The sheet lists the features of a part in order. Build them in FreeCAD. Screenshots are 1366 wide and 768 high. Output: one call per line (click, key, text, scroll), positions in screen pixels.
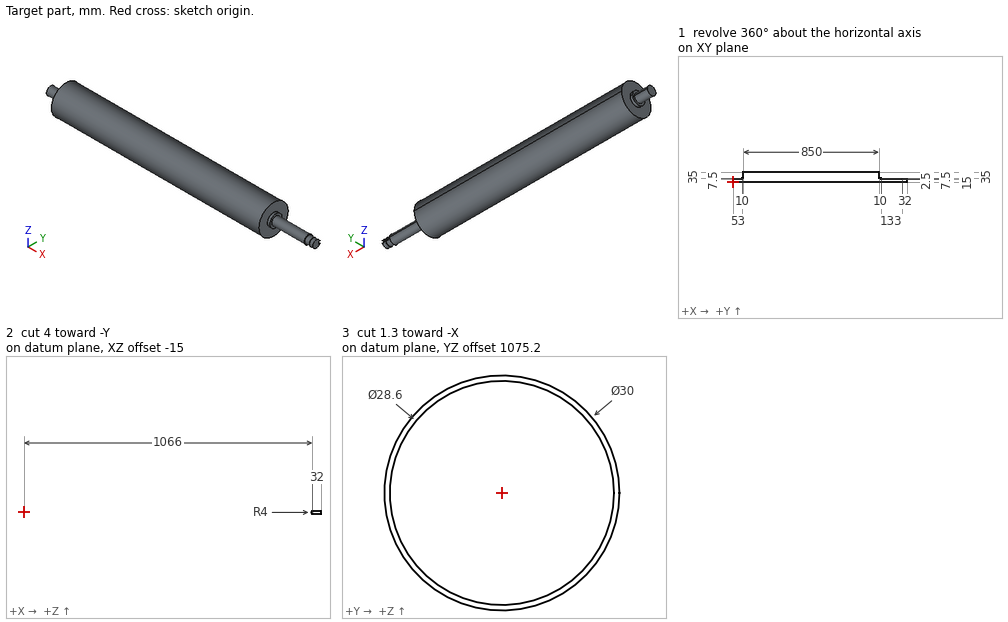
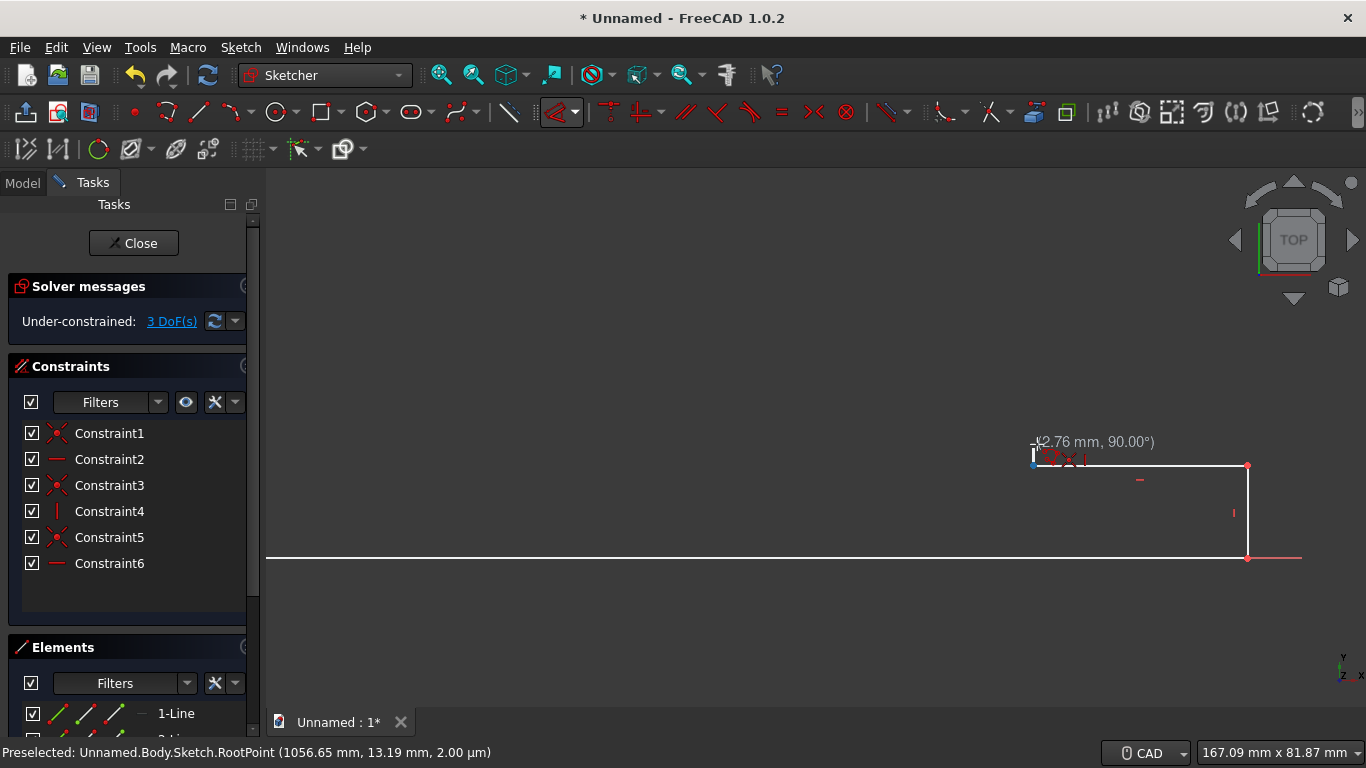
click(1033, 443)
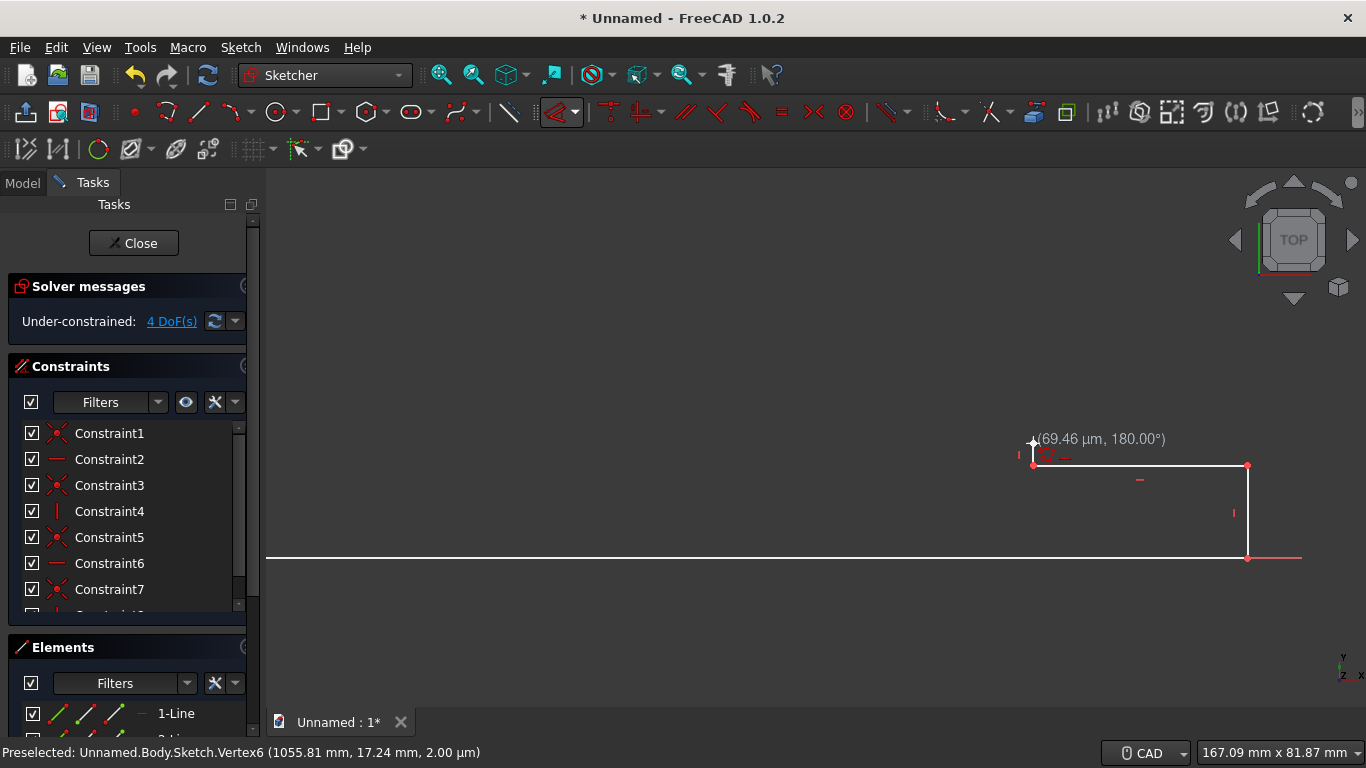
scroll(1055, 445, down, 12)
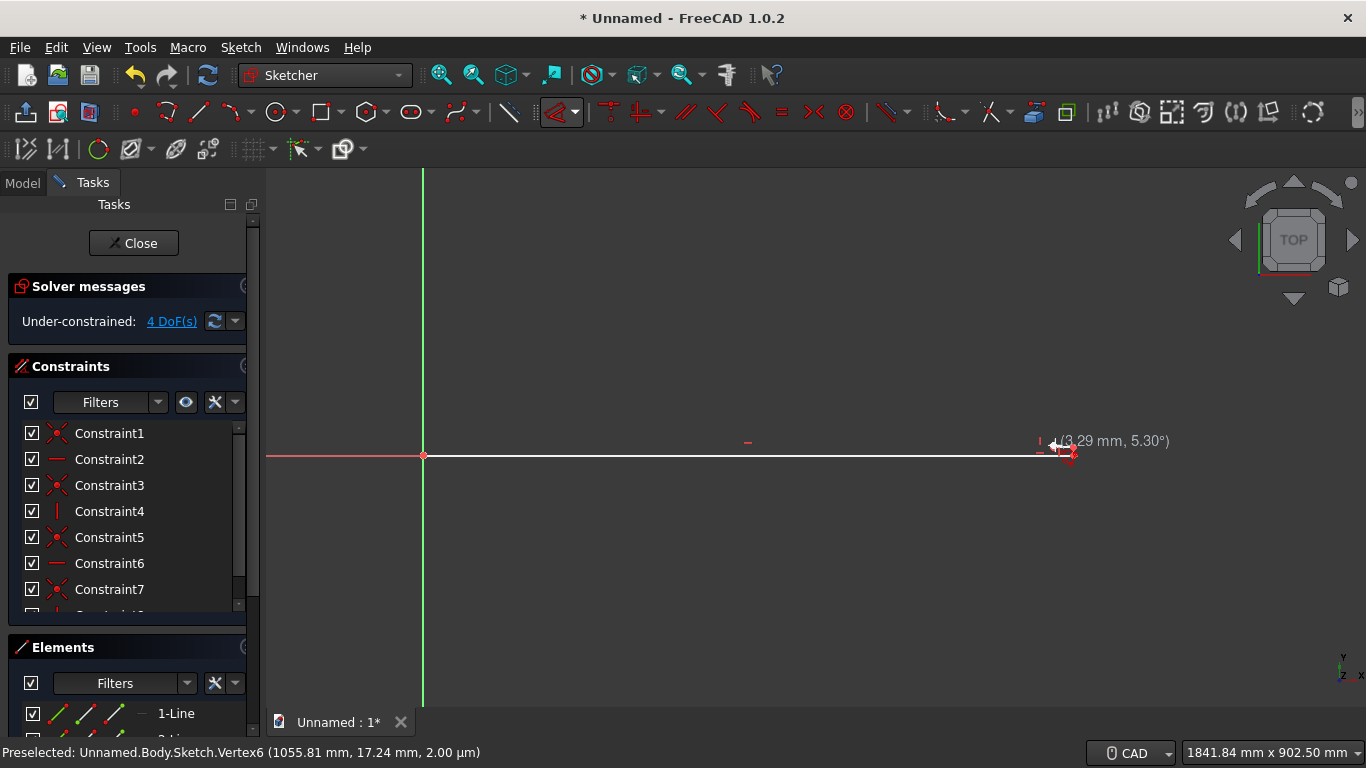
scroll(974, 445, up, 3)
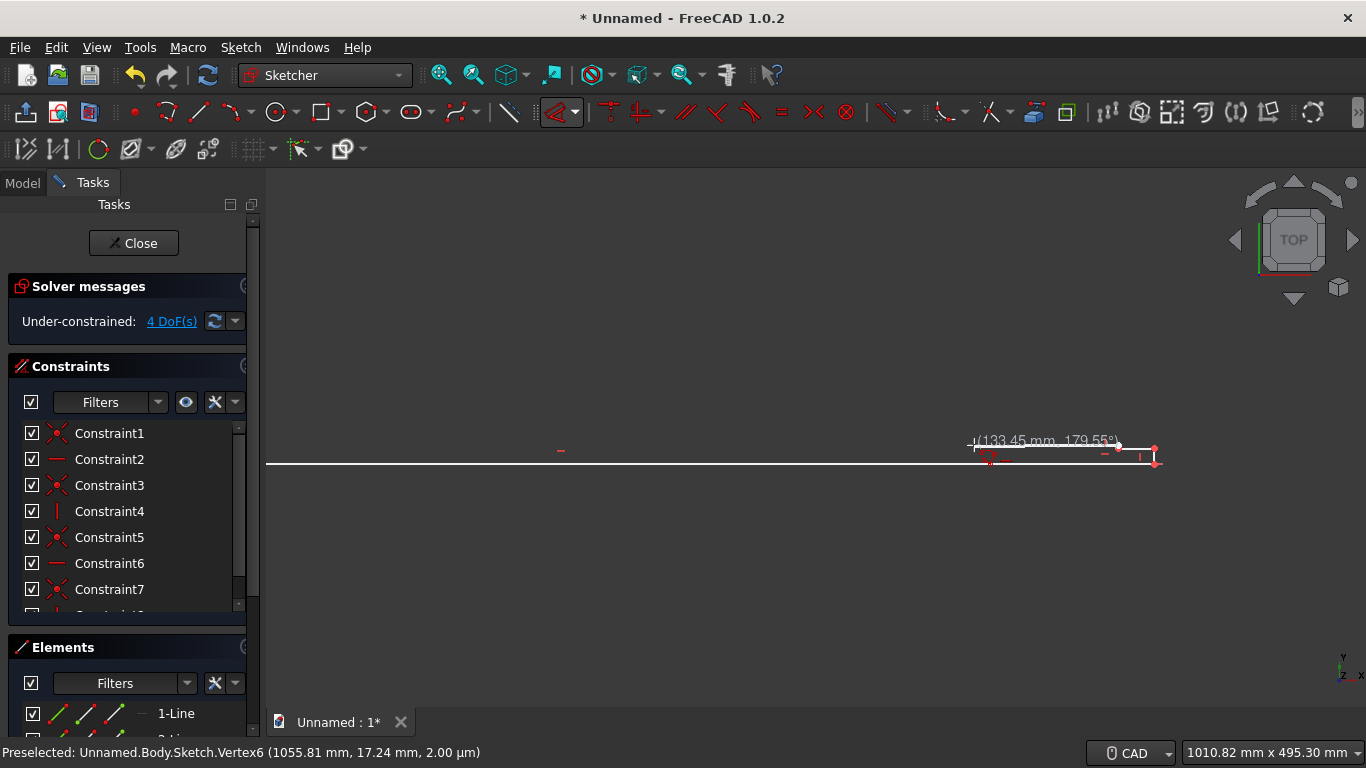
click(974, 445)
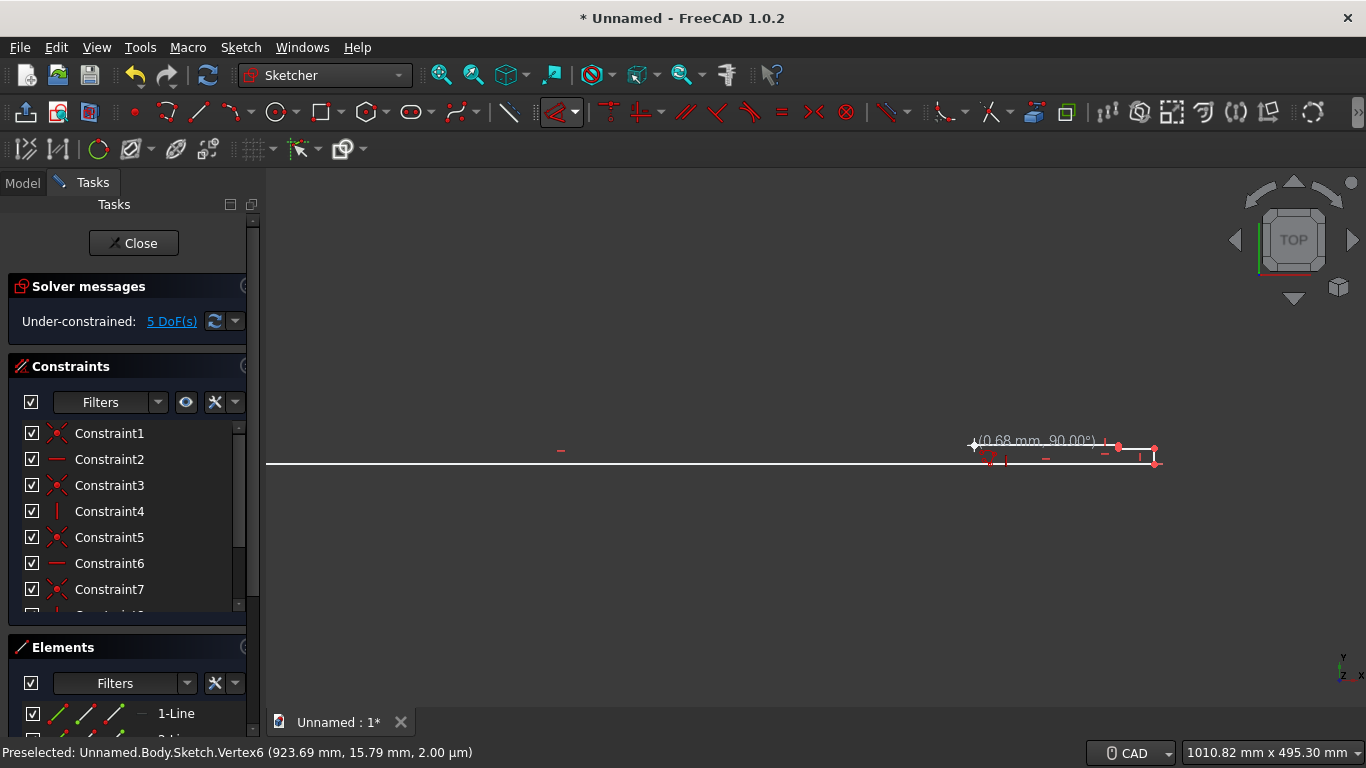
scroll(974, 437, up, 4)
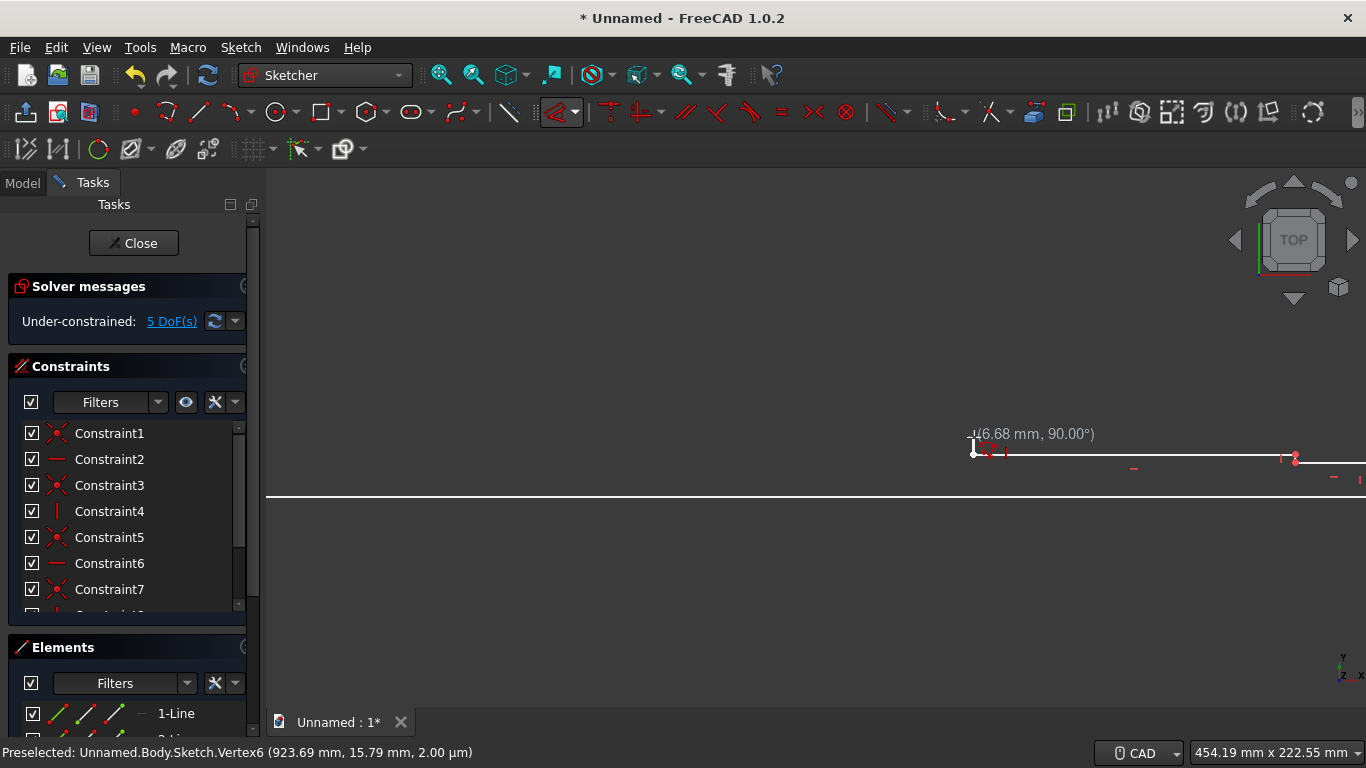
click(973, 436)
click(950, 436)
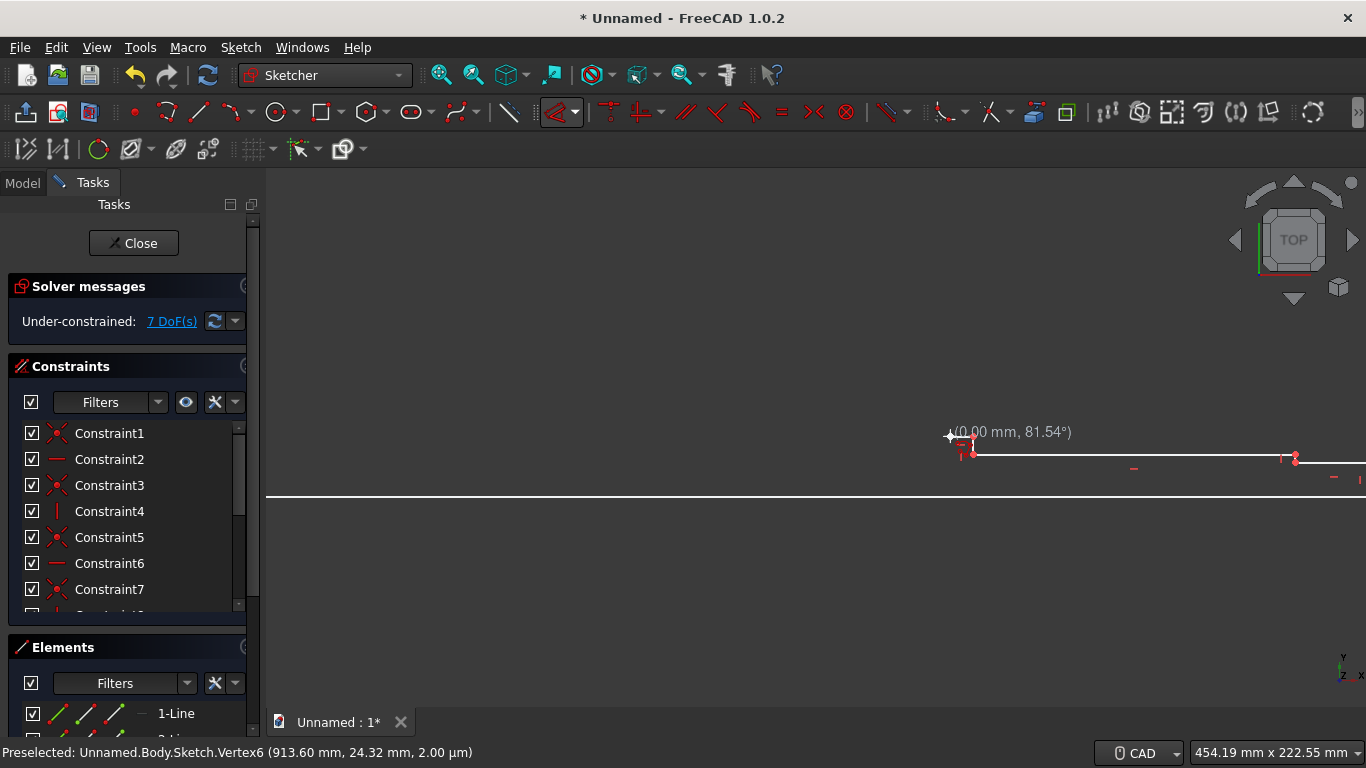
scroll(974, 442, down, 7)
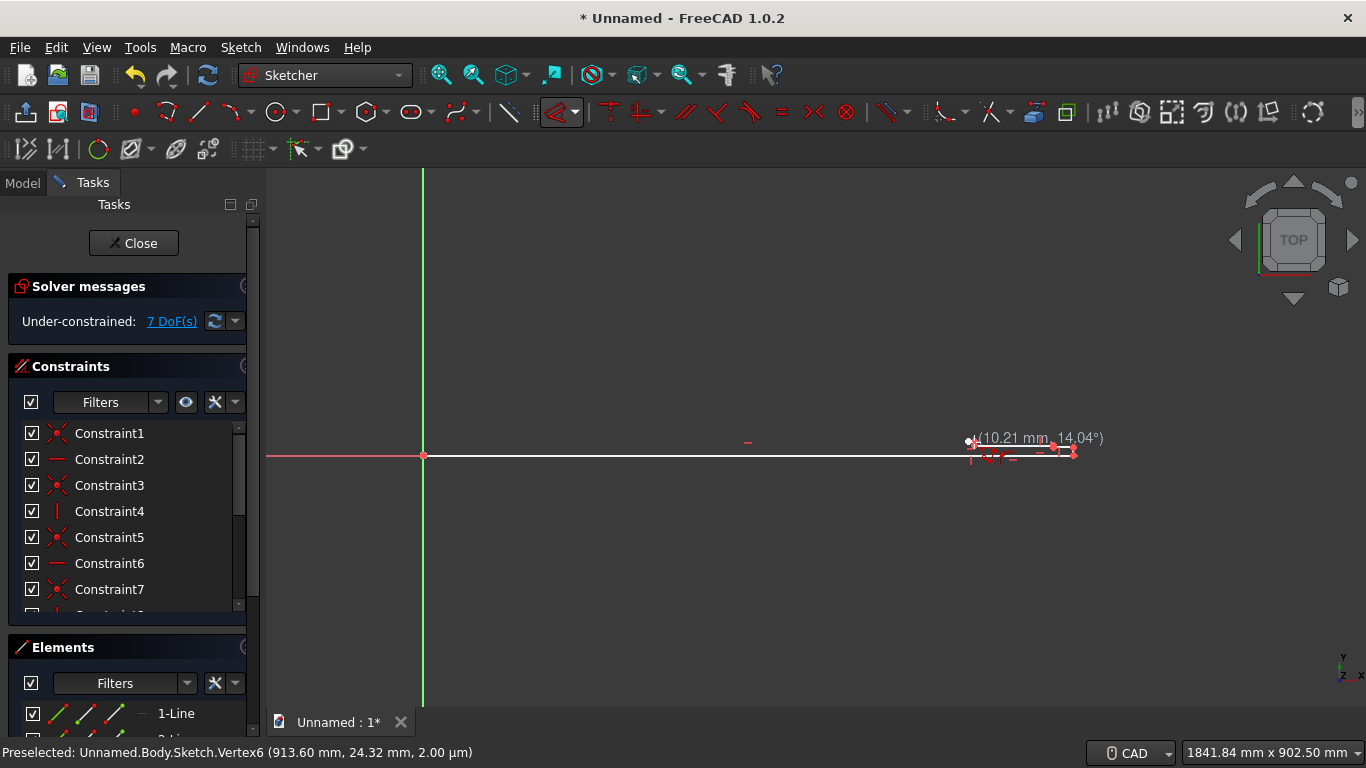
click(969, 420)
click(461, 420)
click(461, 441)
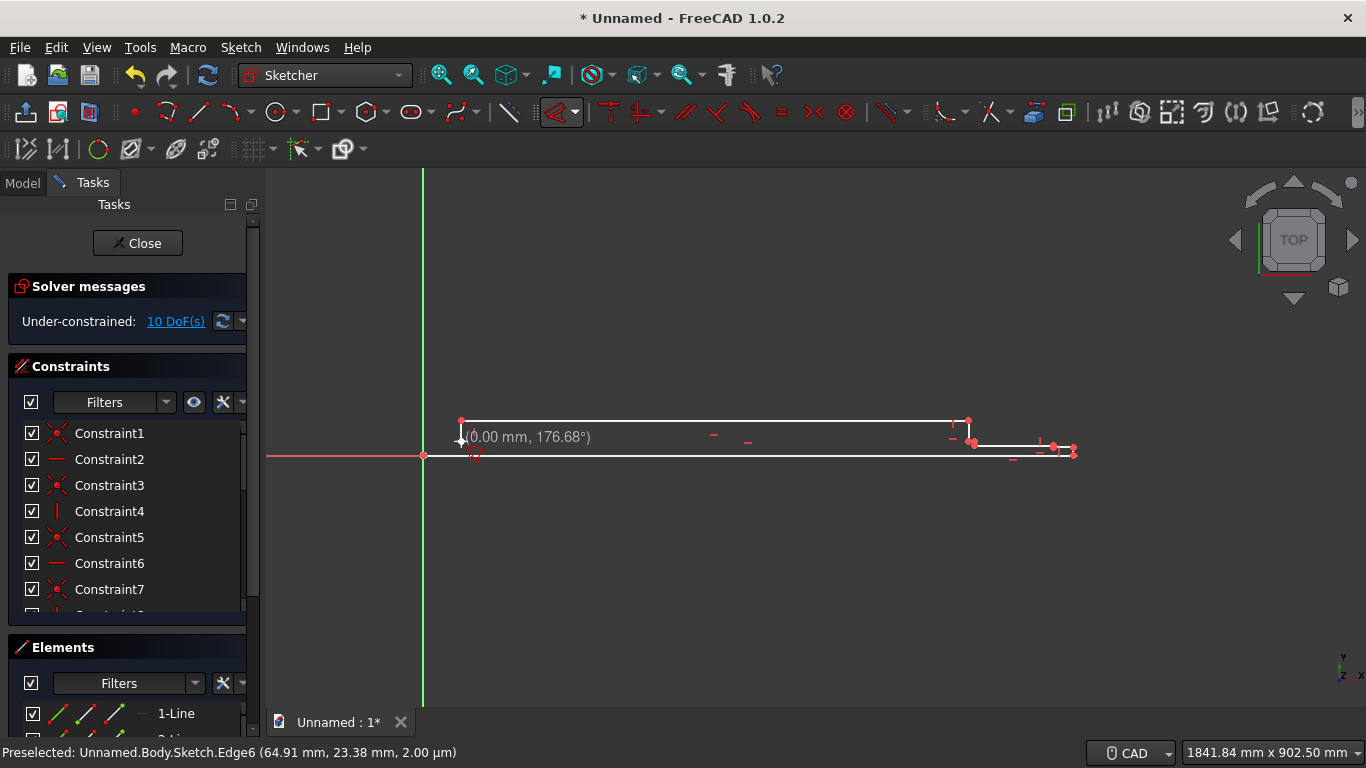
scroll(455, 441, up, 5)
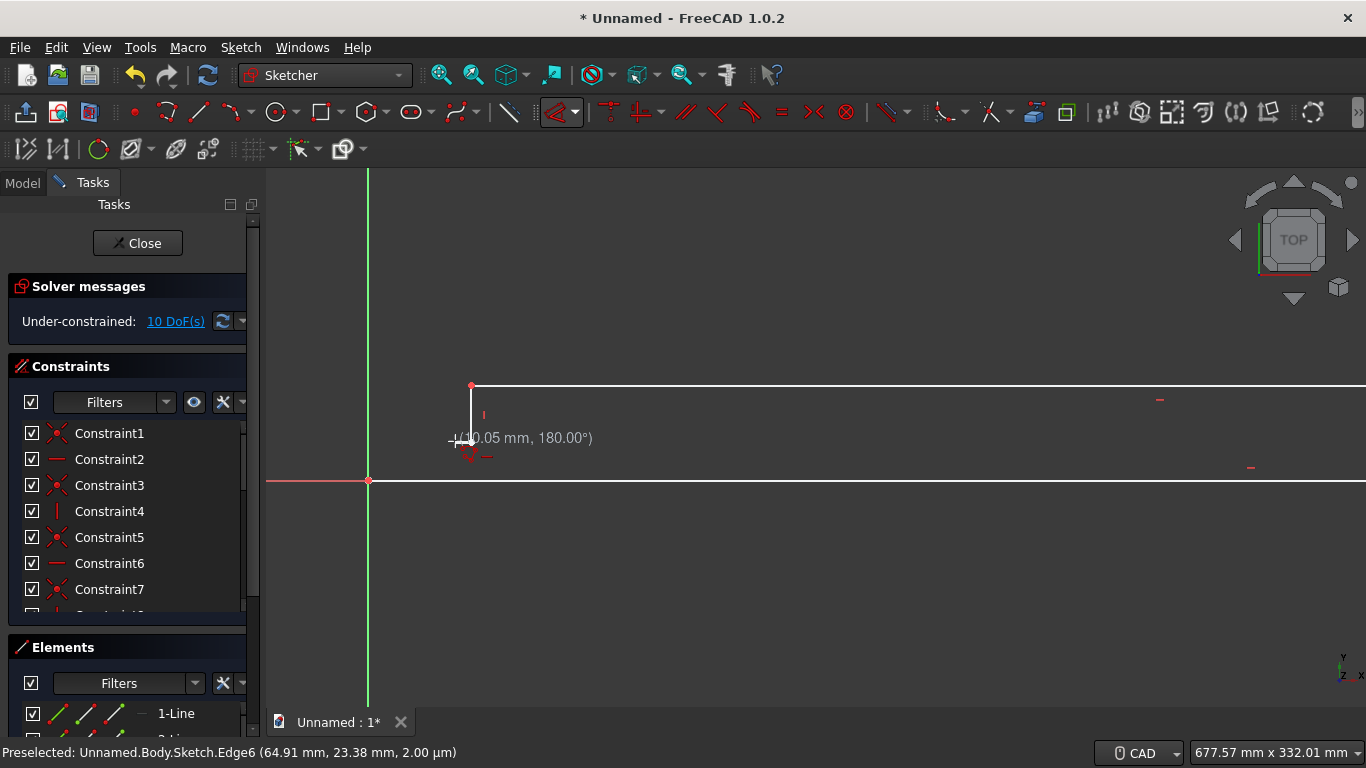
click(454, 440)